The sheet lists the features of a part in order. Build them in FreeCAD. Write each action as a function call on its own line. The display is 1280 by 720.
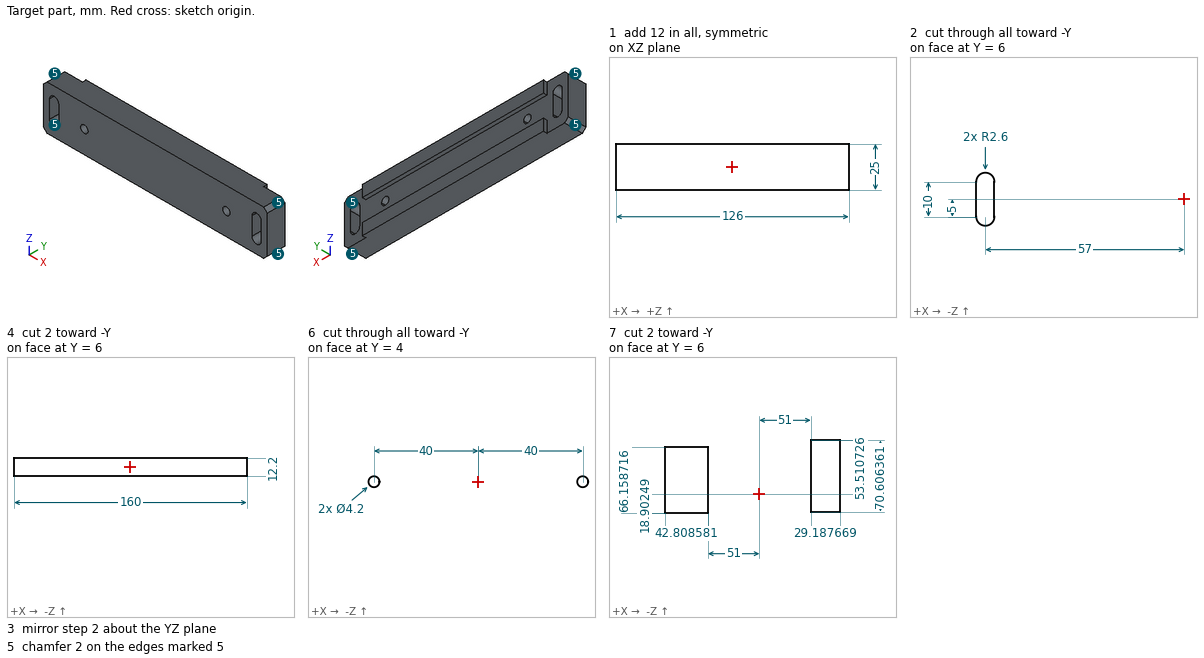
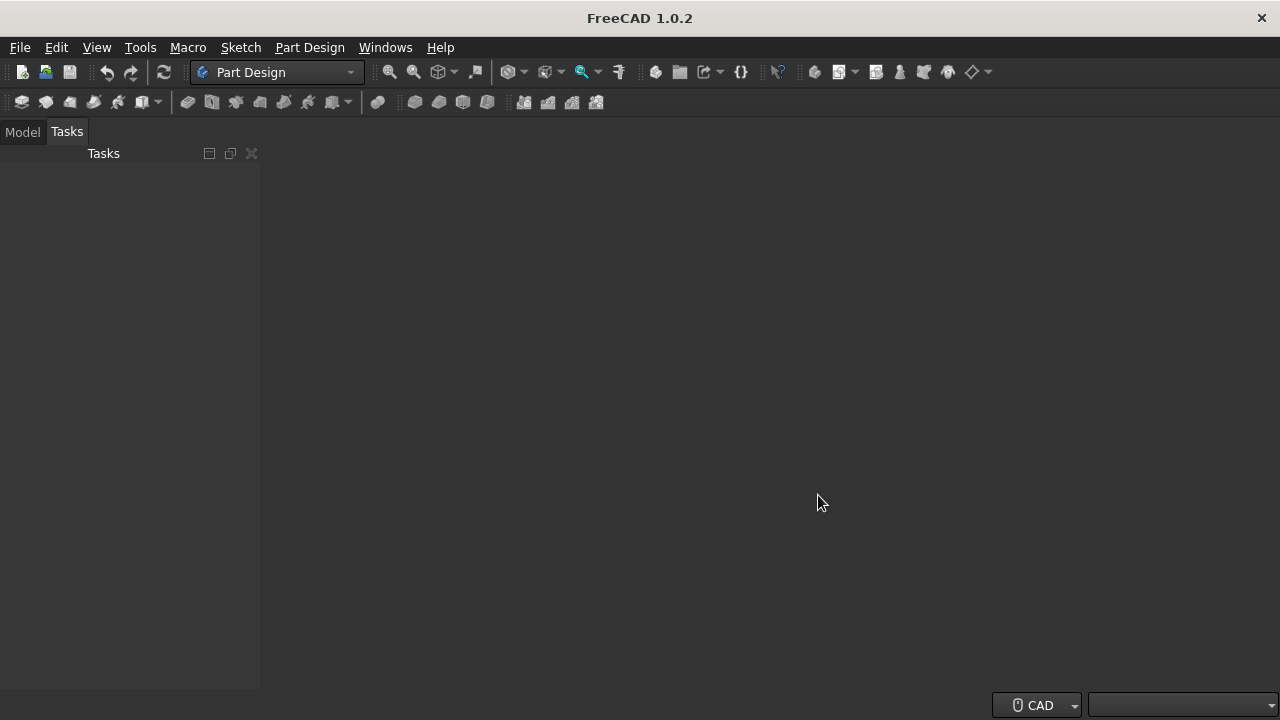
click(22, 72)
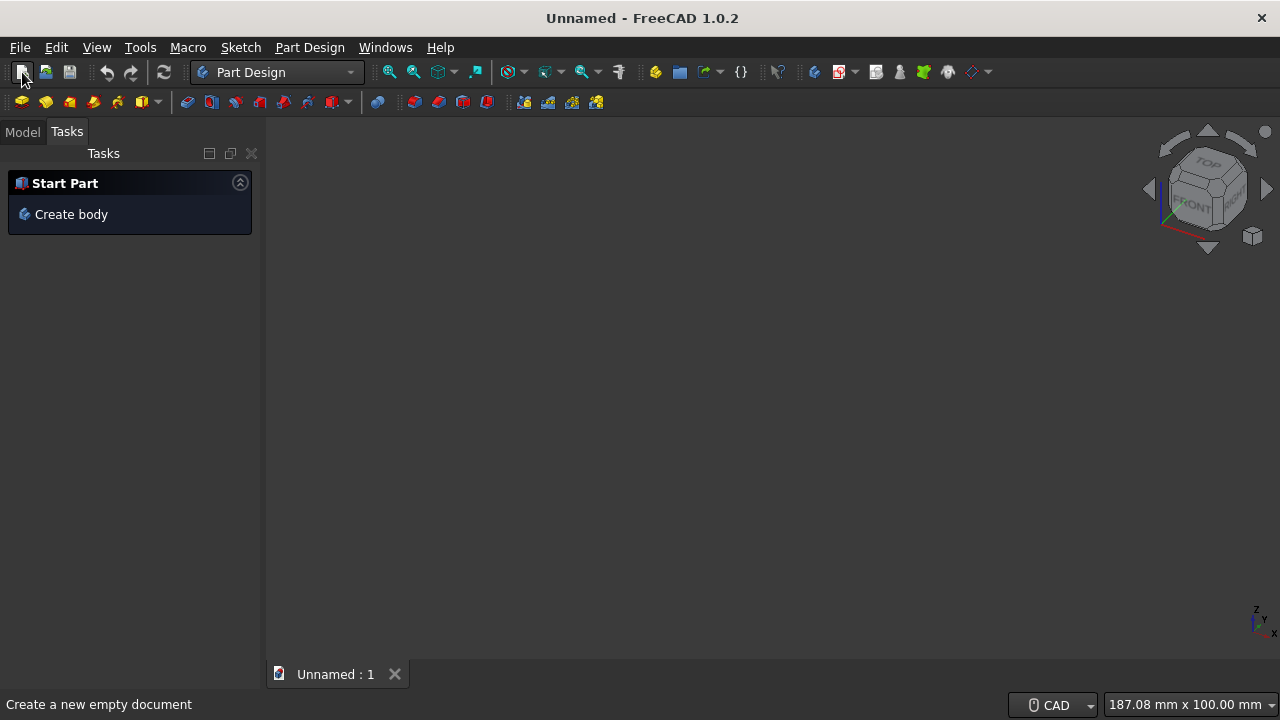
click(840, 72)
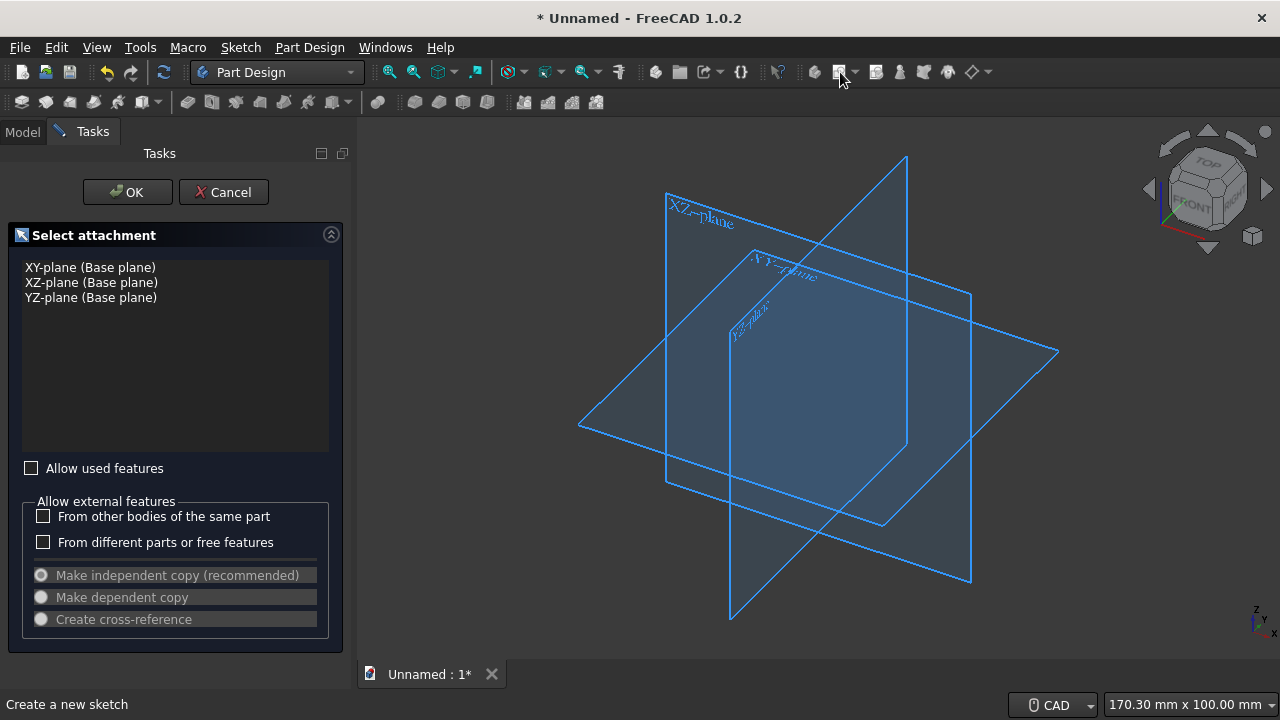
click(82, 282)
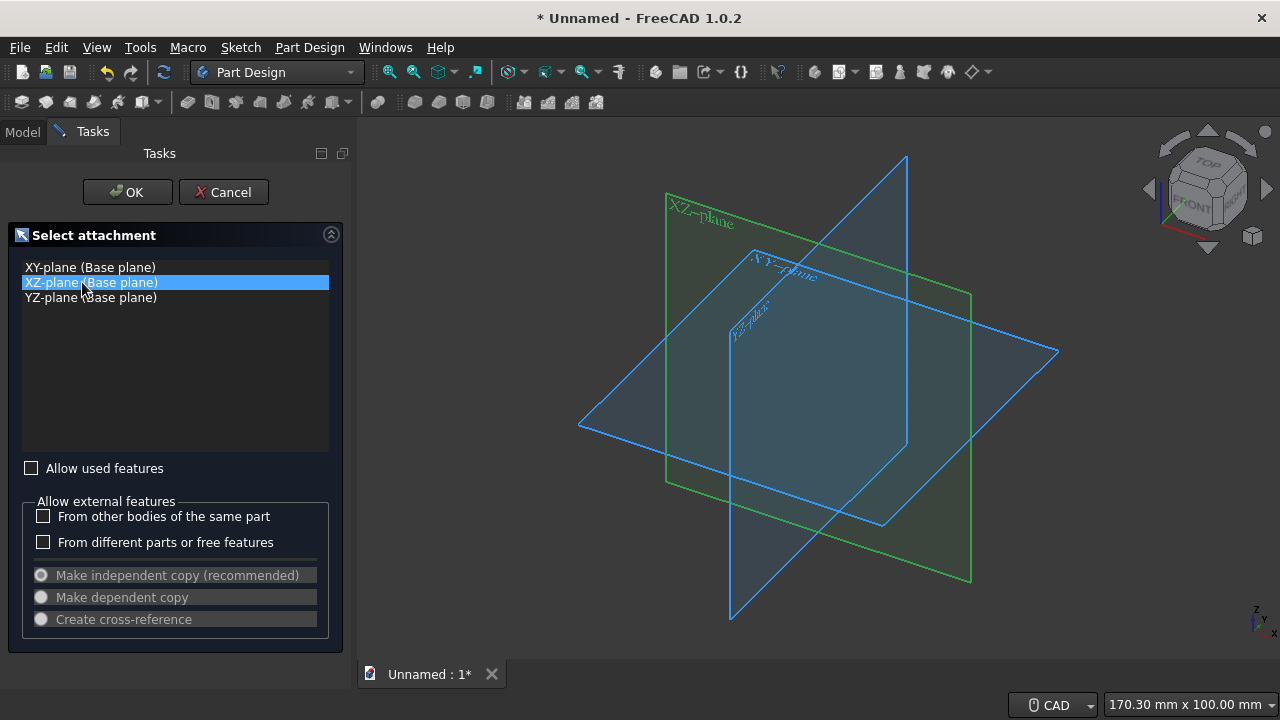
click(128, 192)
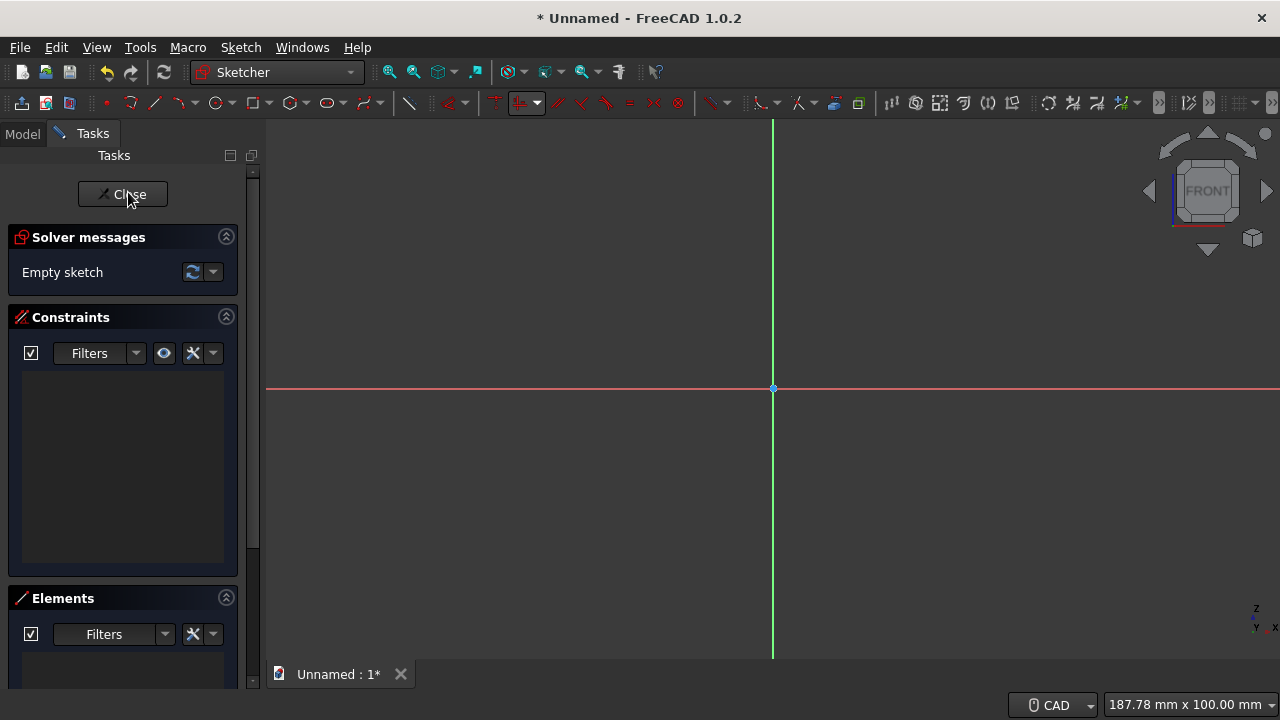
scroll(395, 389, down, 1)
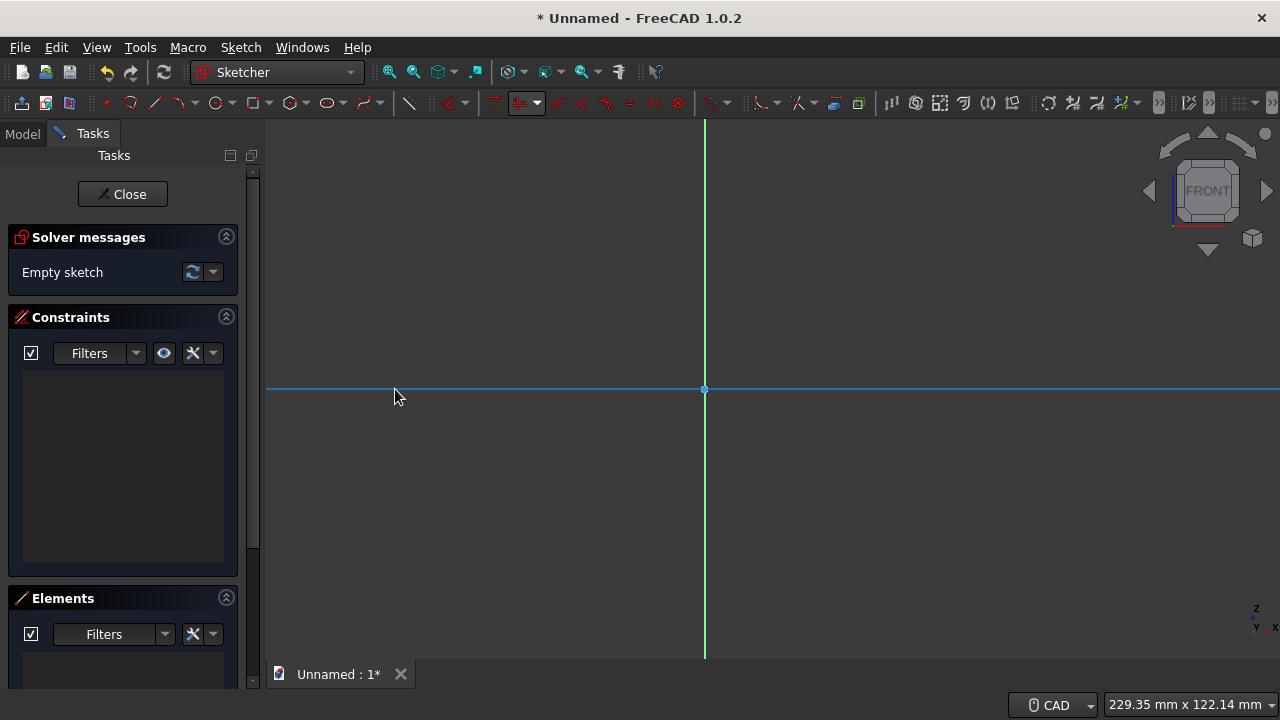
key(g)
key(v)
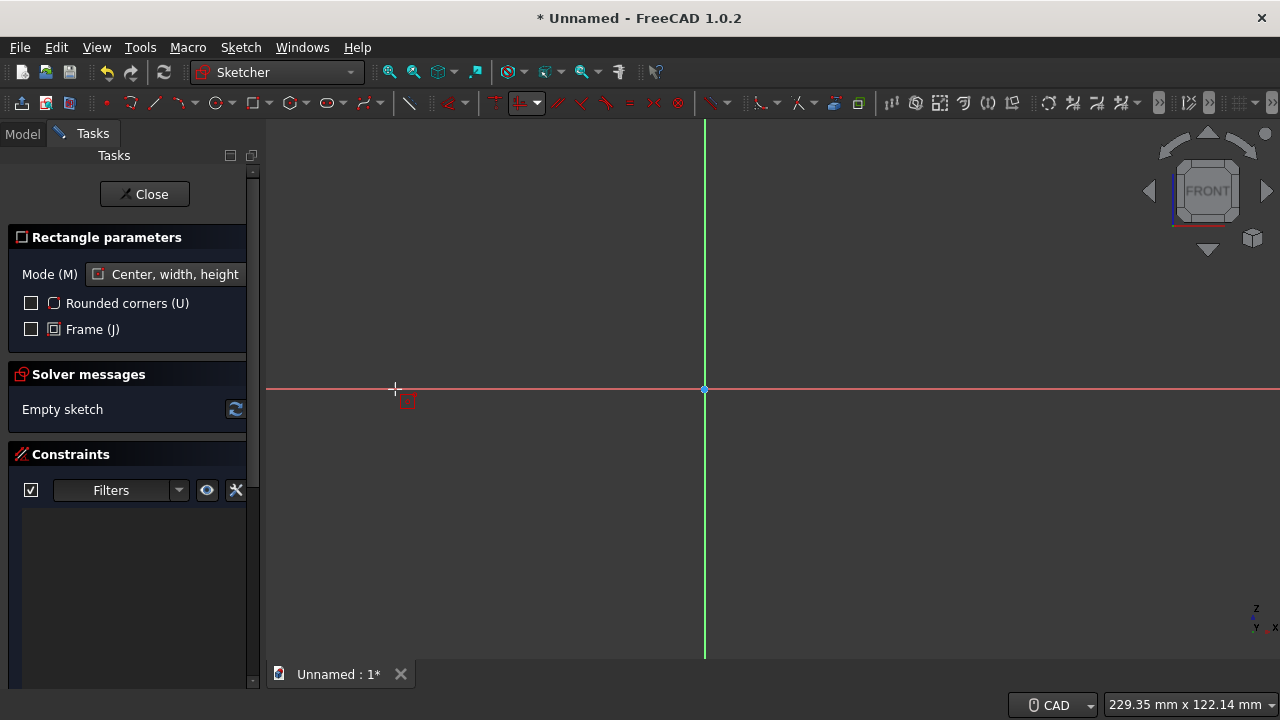
click(705, 389)
click(983, 334)
key(Escape)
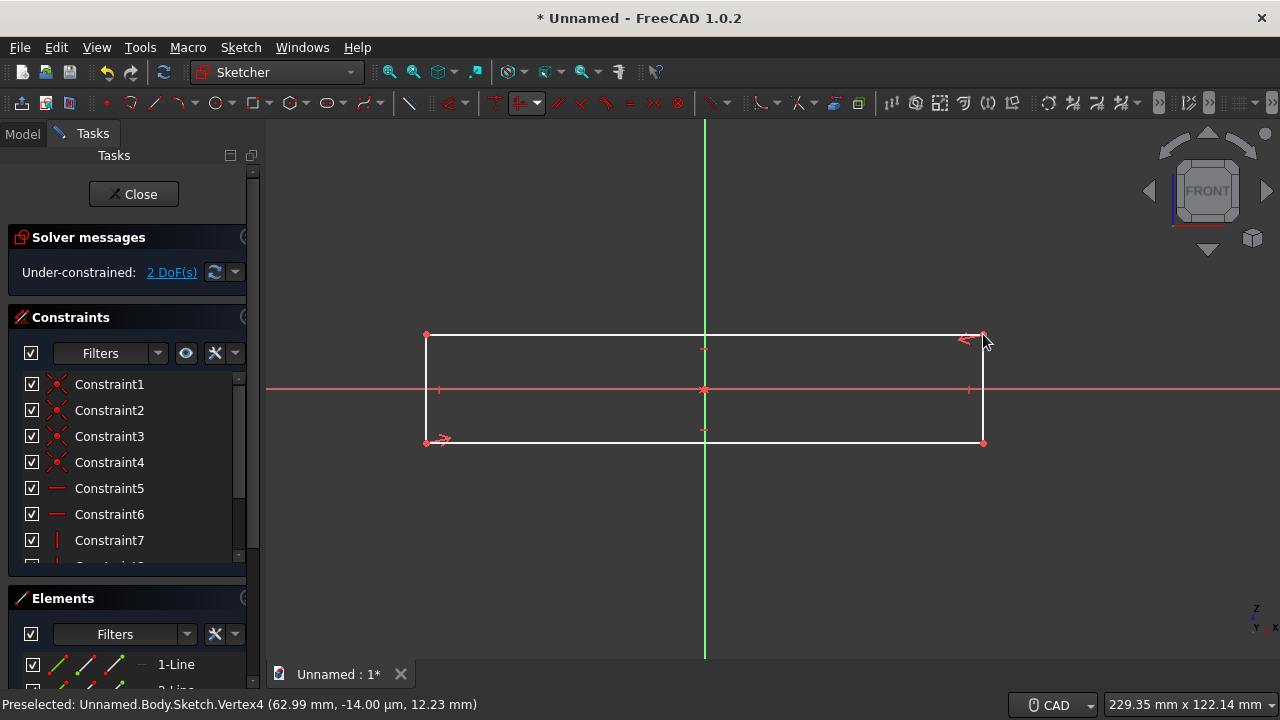
click(448, 104)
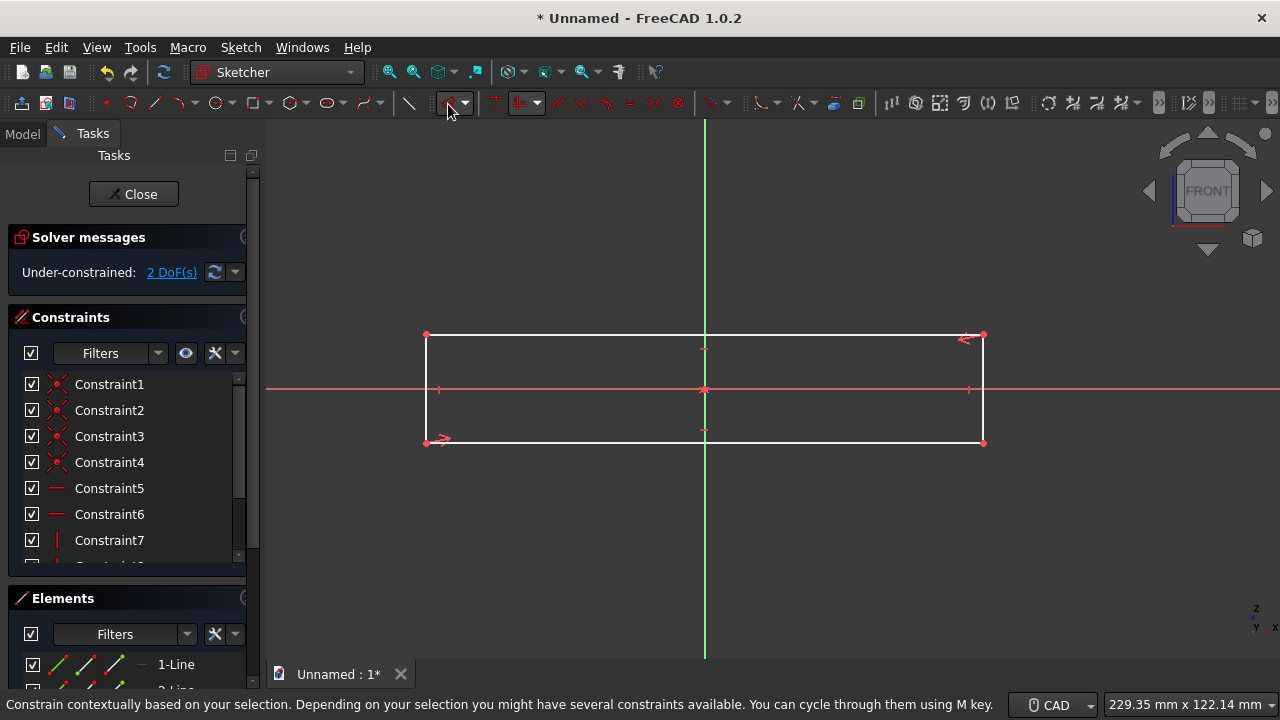
click(983, 411)
click(1017, 364)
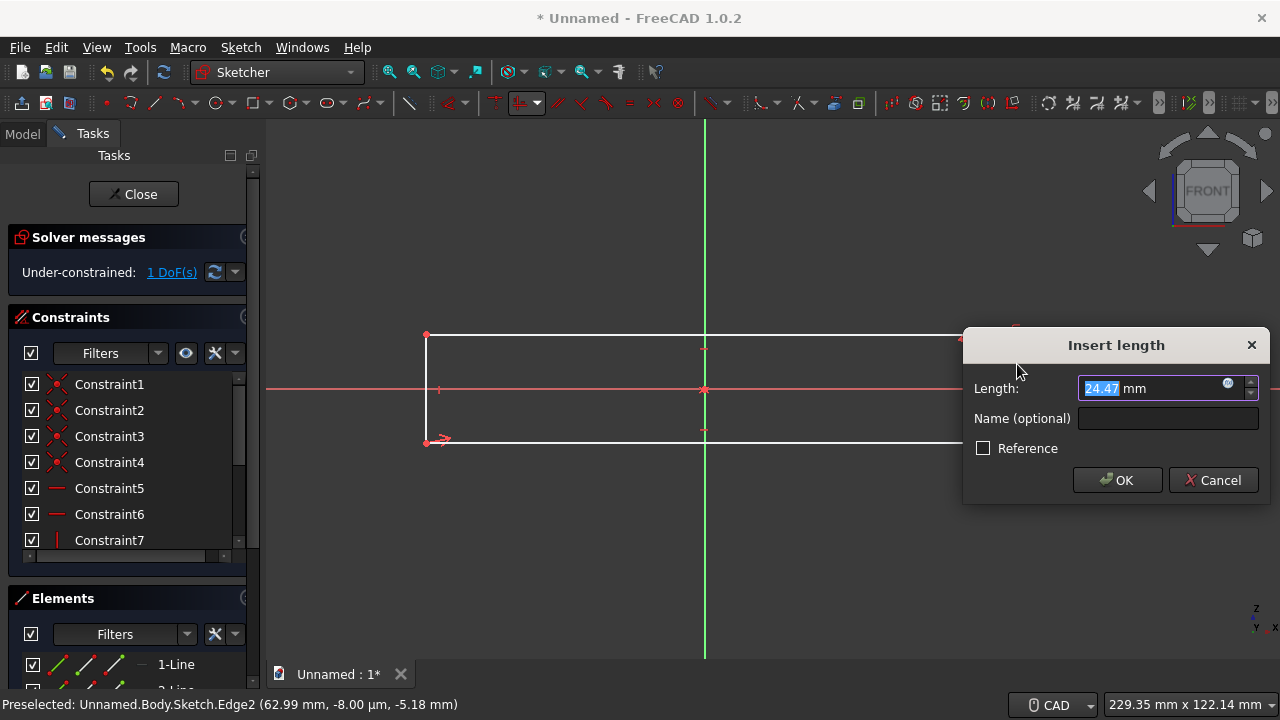
text(25)
key(Return)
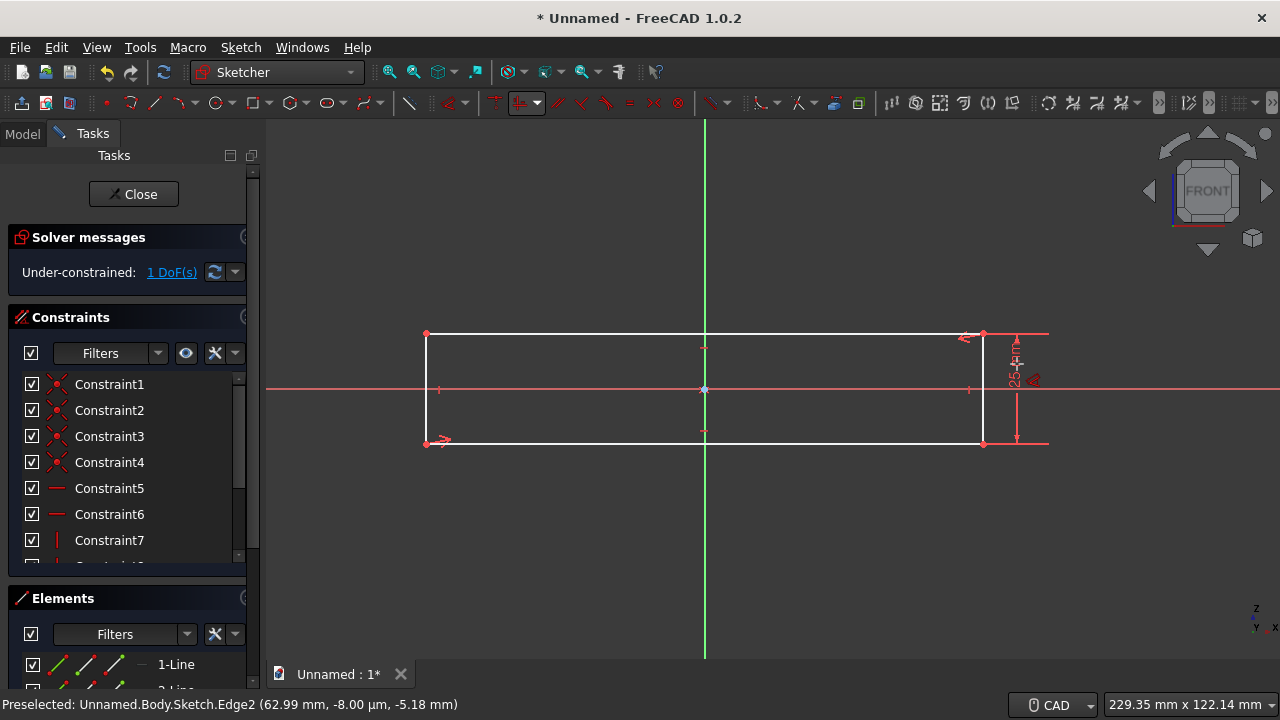
click(593, 444)
click(576, 478)